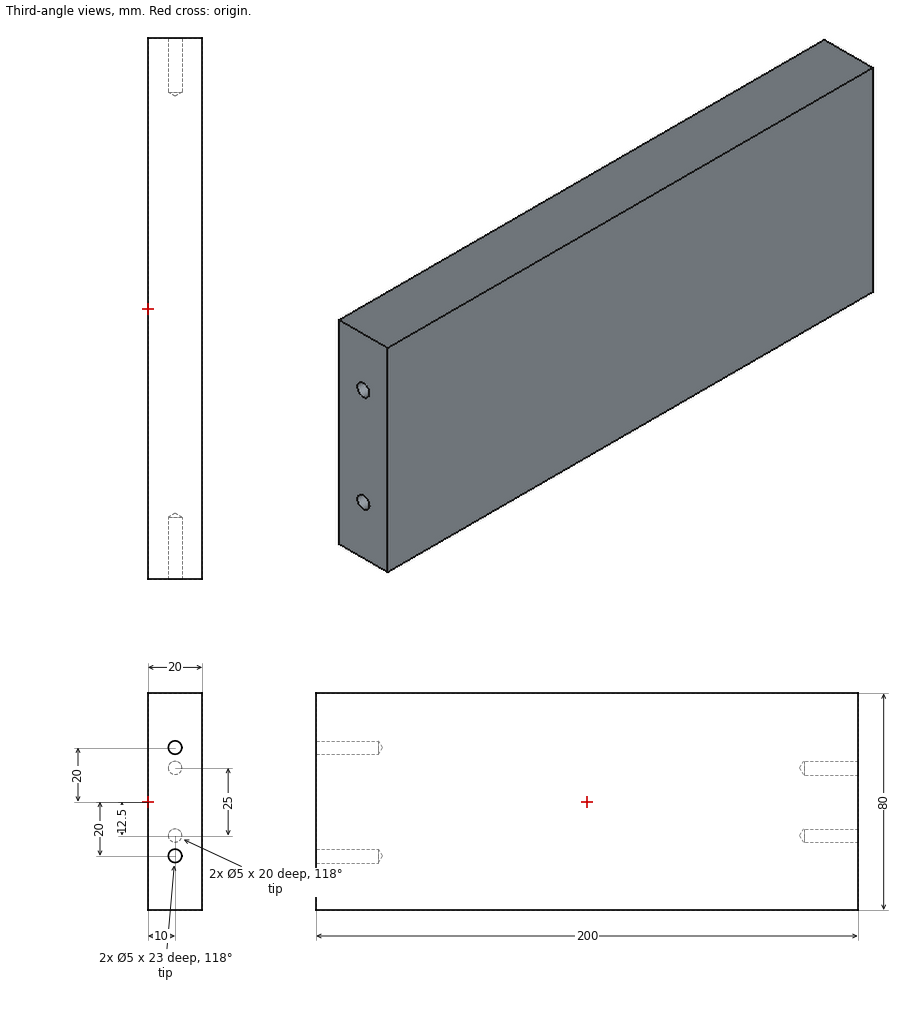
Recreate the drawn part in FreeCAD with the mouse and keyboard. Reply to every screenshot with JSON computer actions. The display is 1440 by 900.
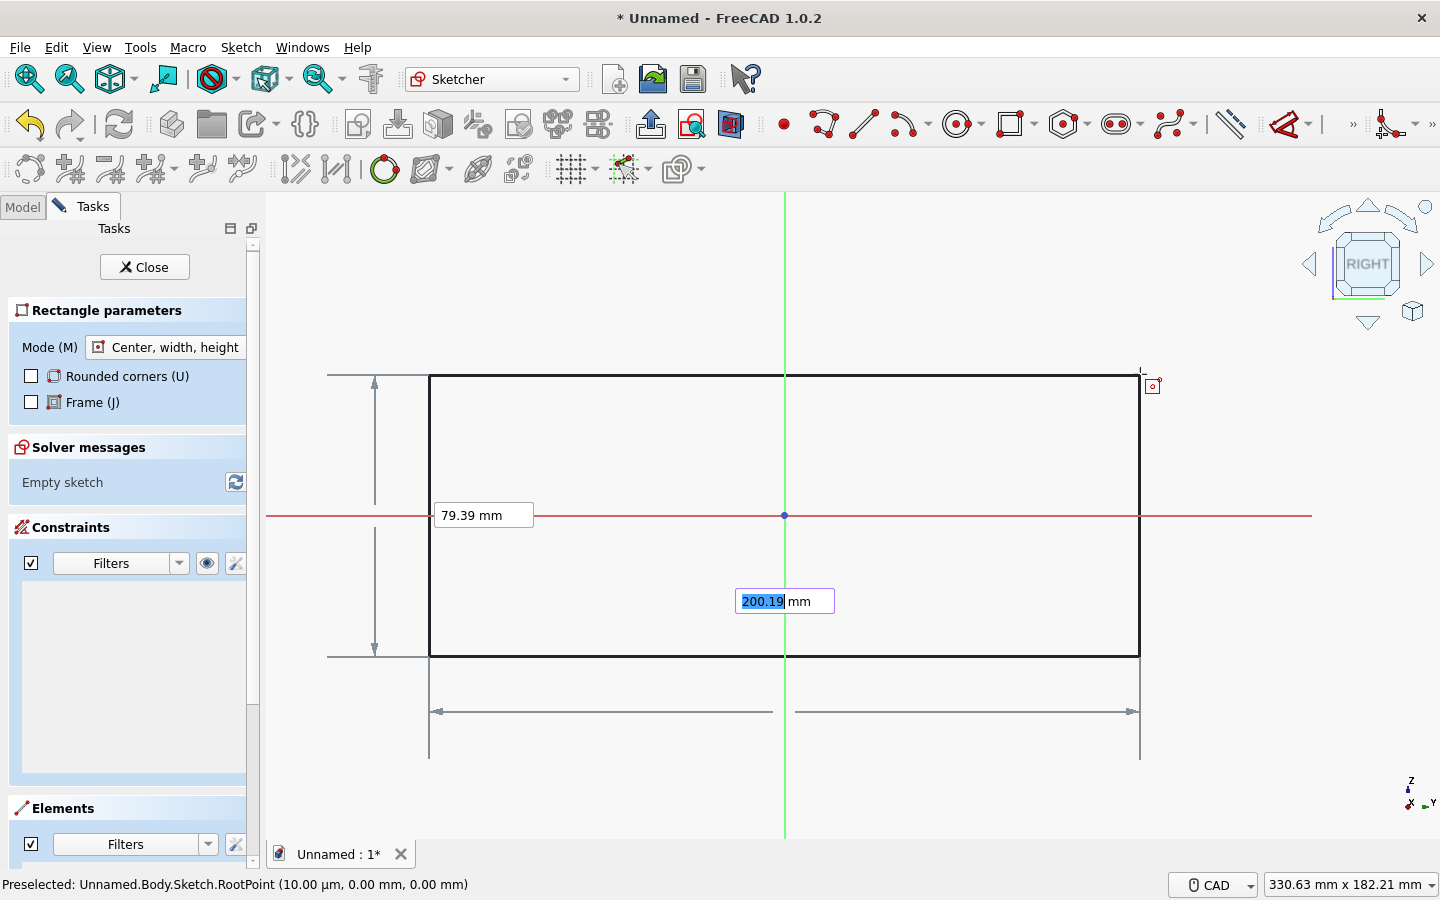
{"action": "type", "text": "200"}
{"action": "key", "text": "Tab"}
{"action": "type", "text": "80"}
{"action": "key", "text": "Return"}
{"action": "key", "text": "Escape"}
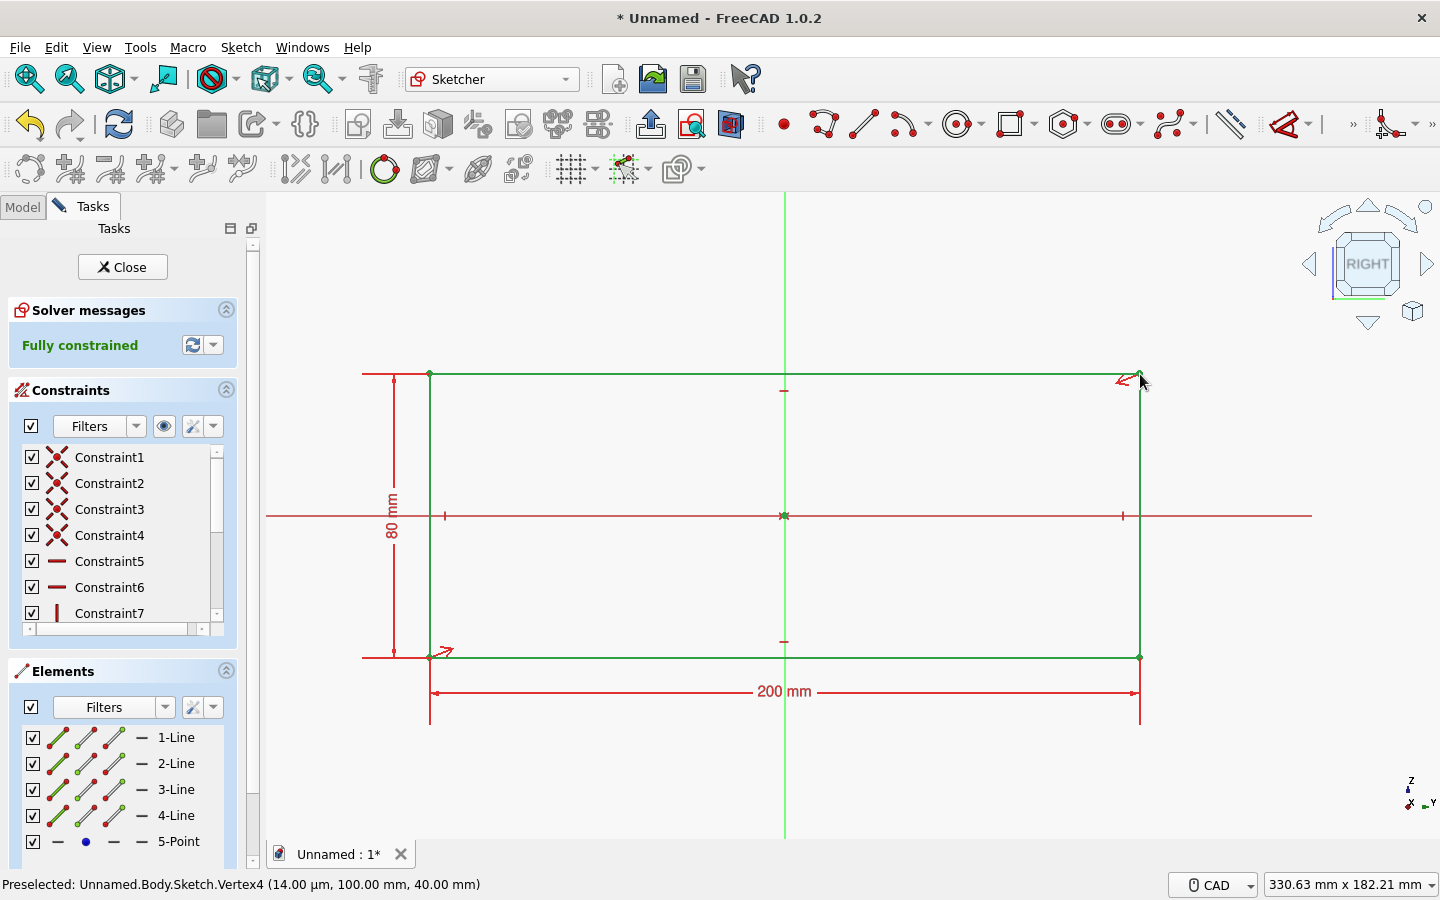
{"action": "left_click", "coordinate": [123, 267]}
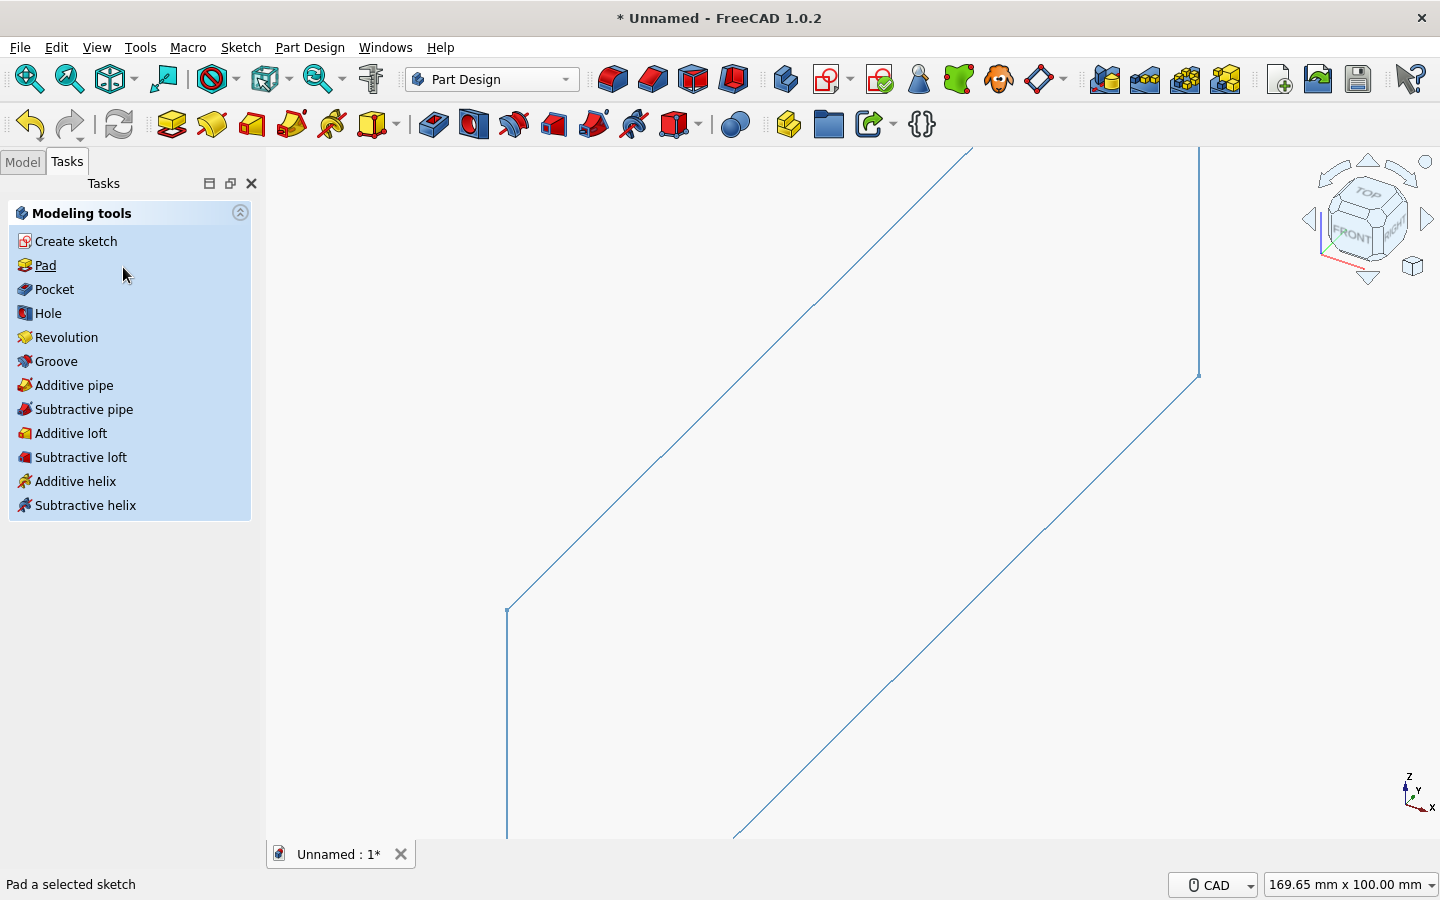
{"action": "left_click", "coordinate": [172, 124]}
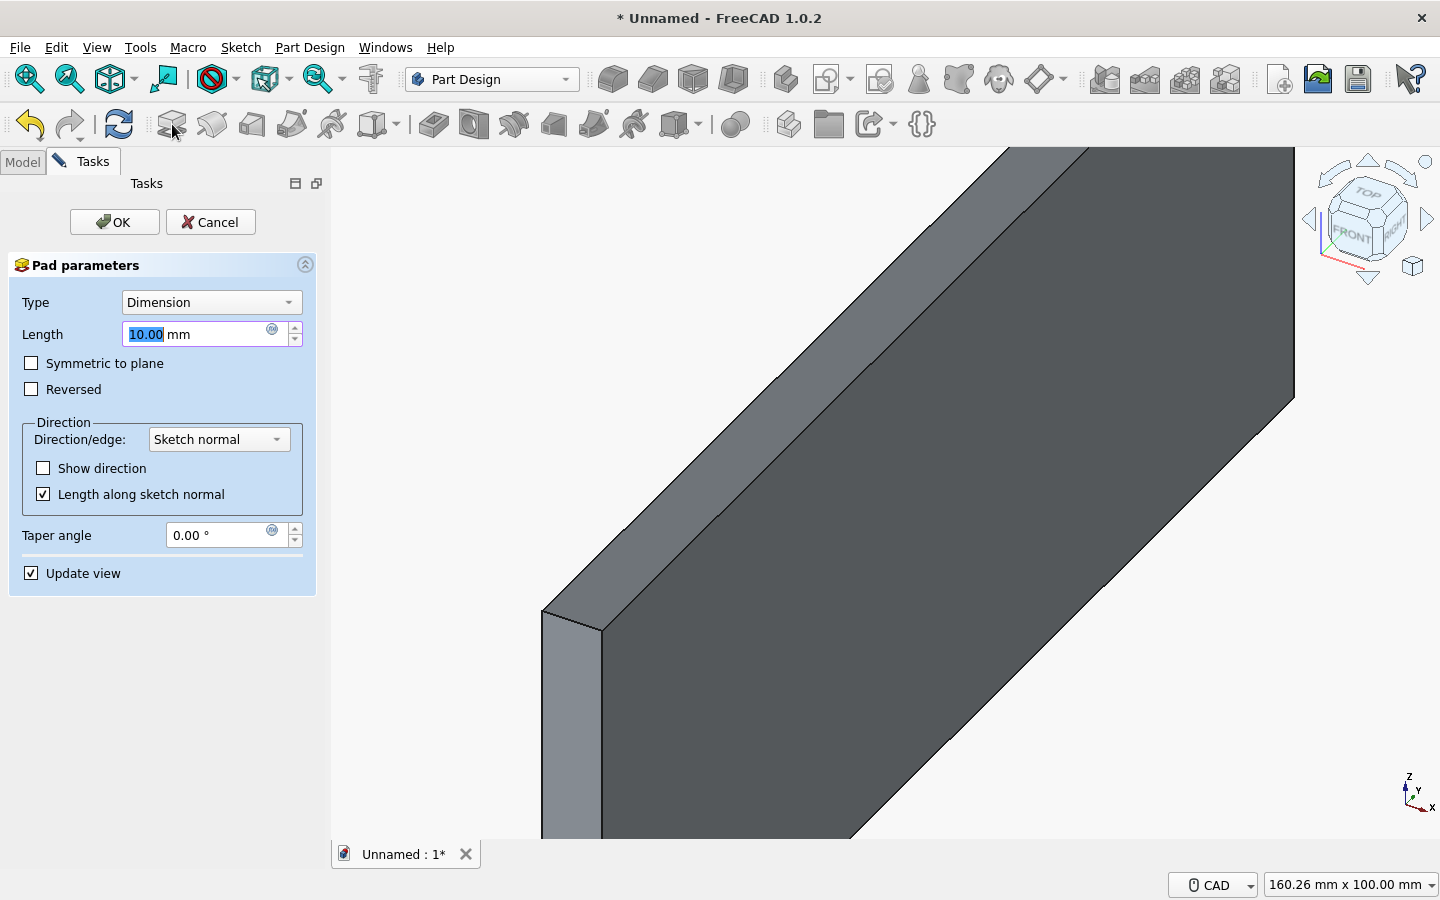
{"action": "type", "text": "20"}
{"action": "key", "text": "Tab"}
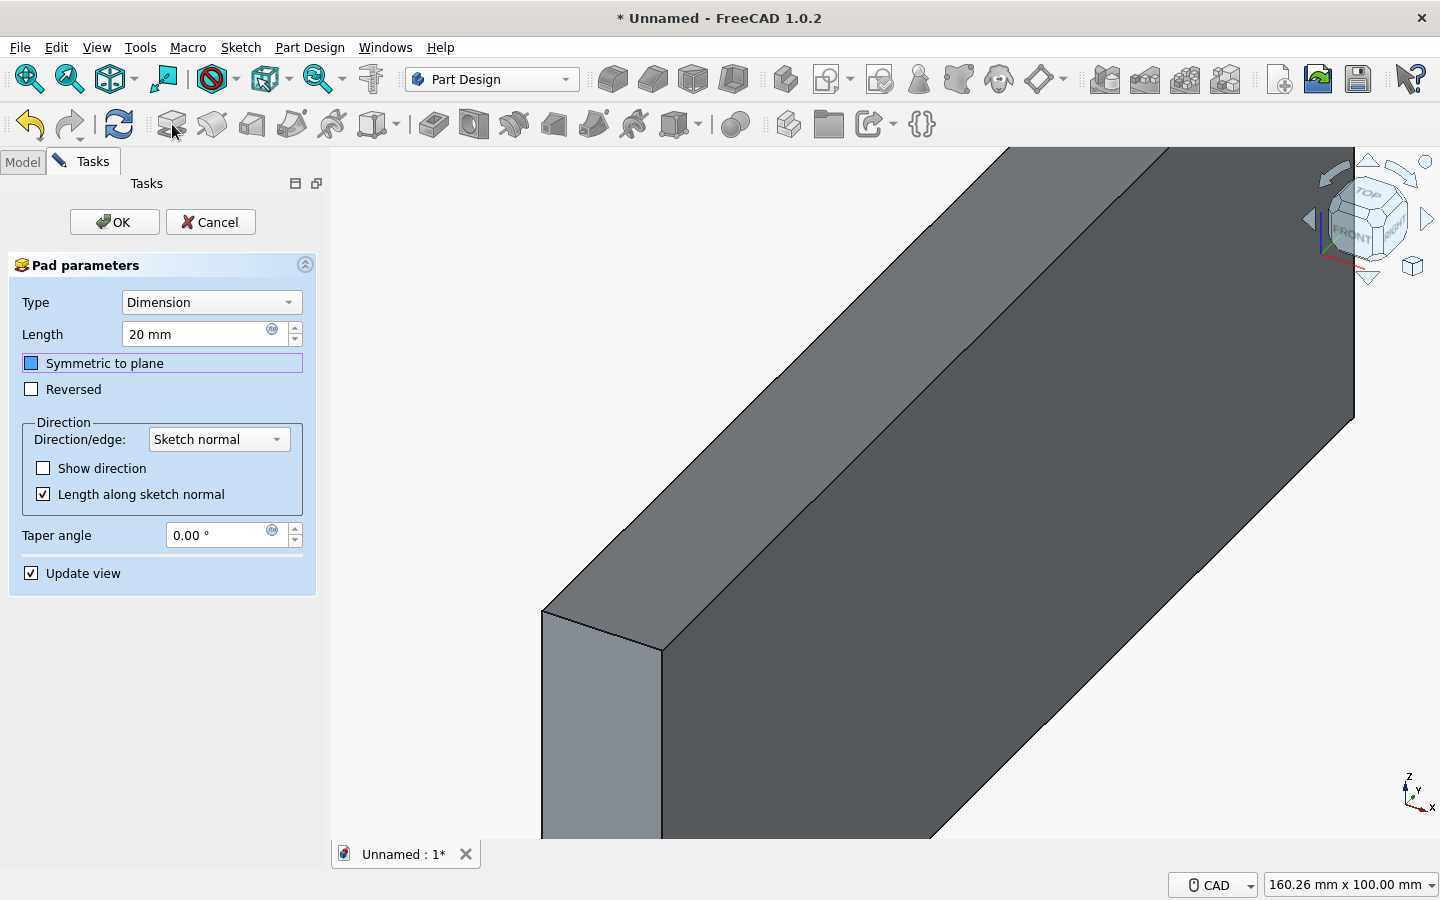
{"action": "left_click", "coordinate": [115, 222]}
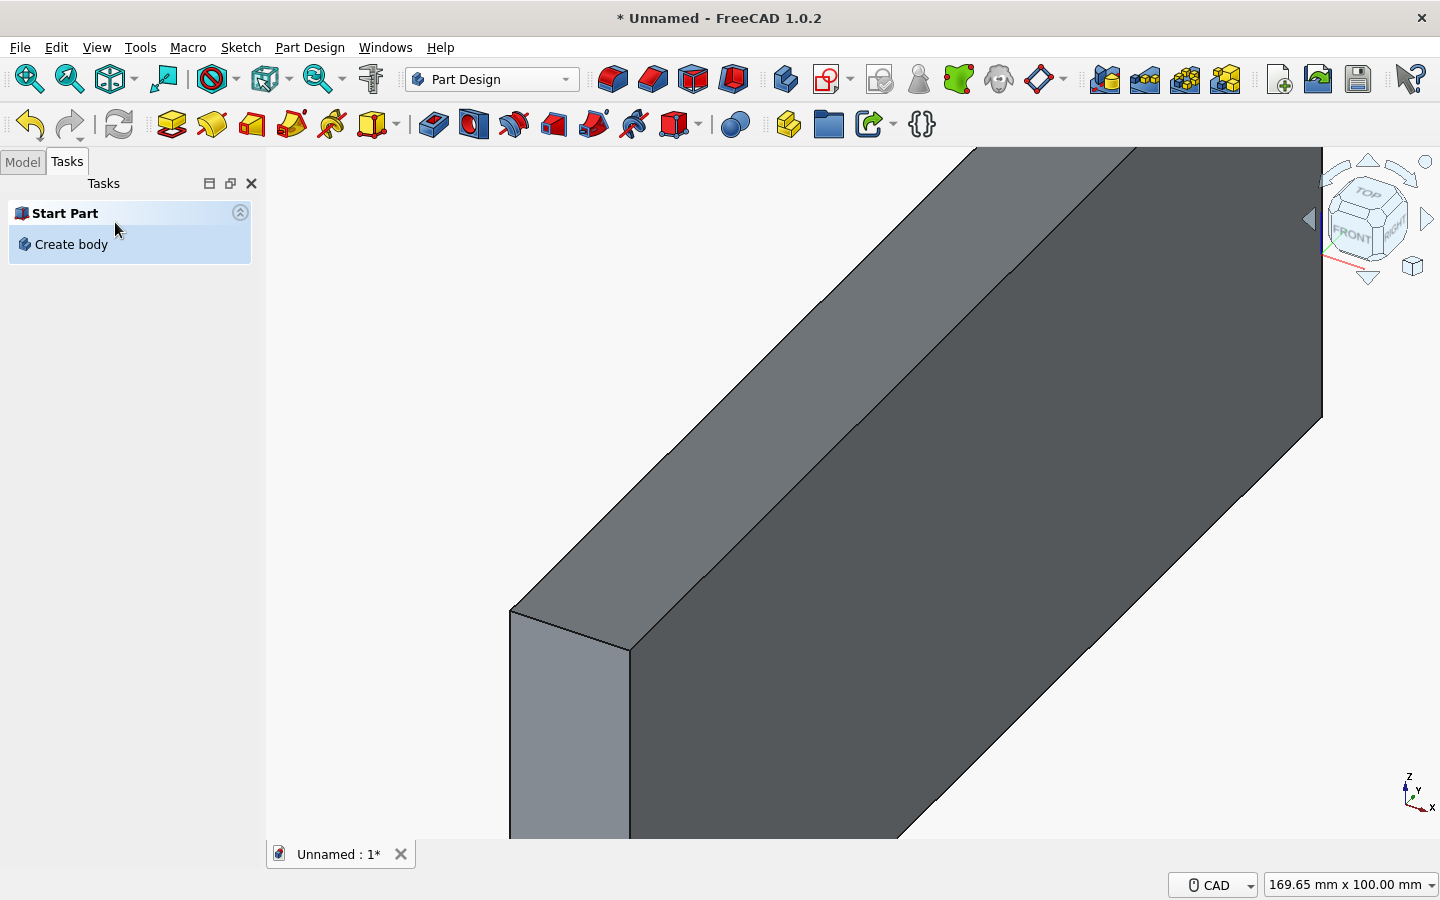
{"action": "left_click", "coordinate": [30, 80]}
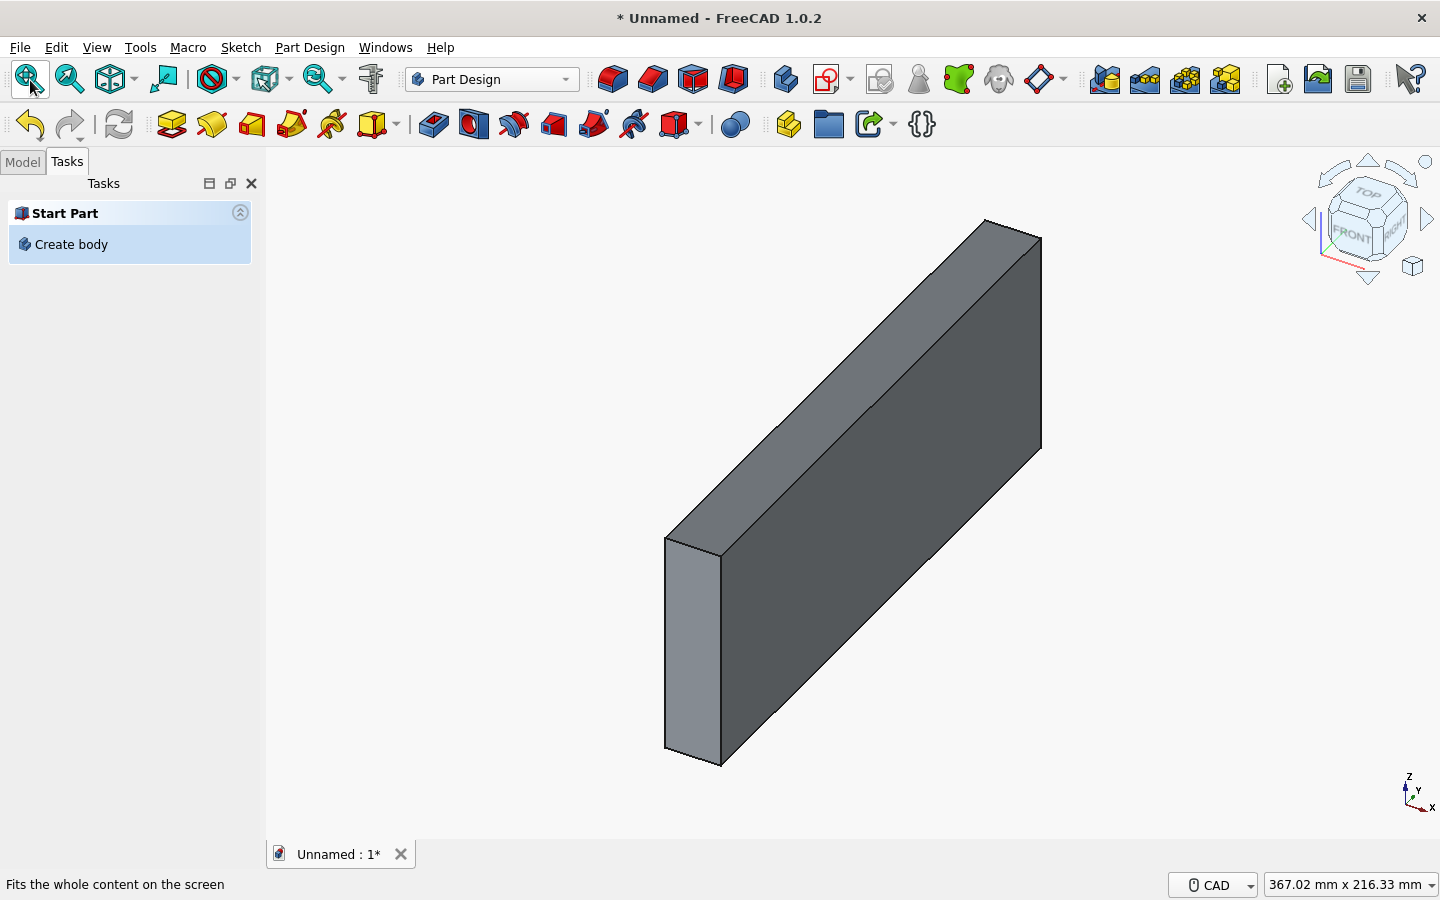
{"action": "key", "text": "4"}